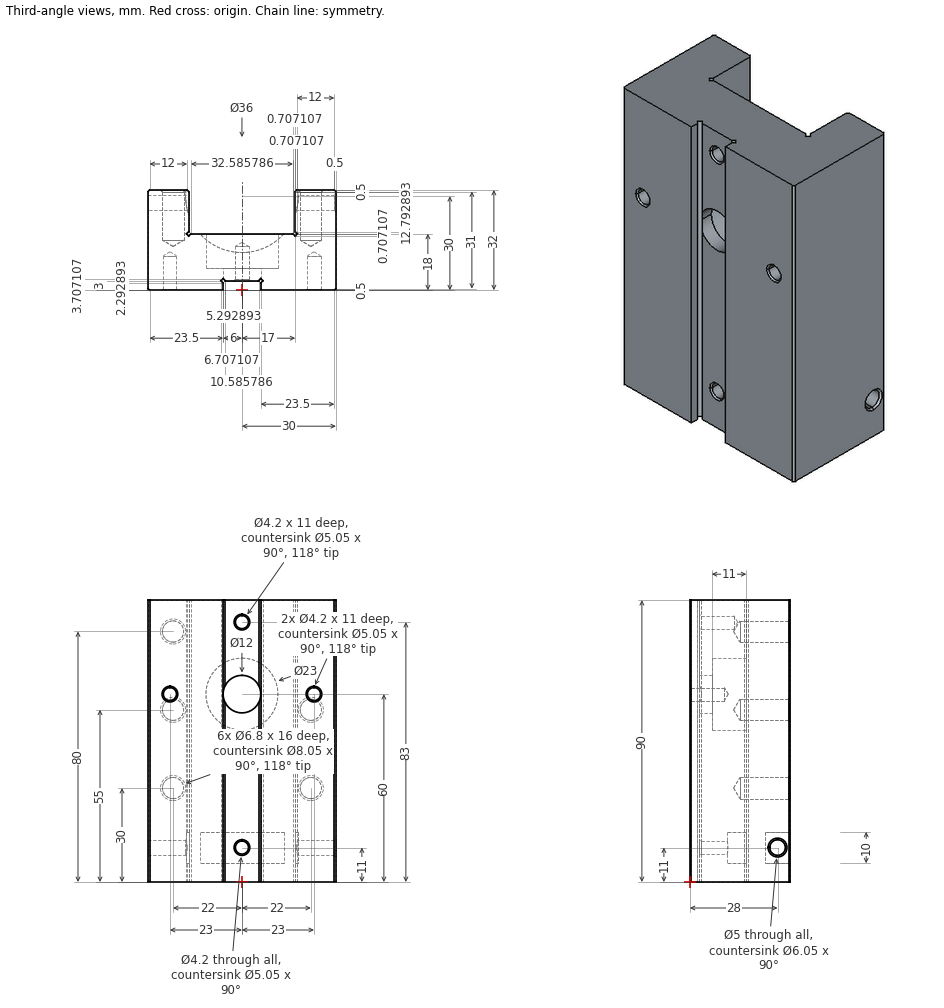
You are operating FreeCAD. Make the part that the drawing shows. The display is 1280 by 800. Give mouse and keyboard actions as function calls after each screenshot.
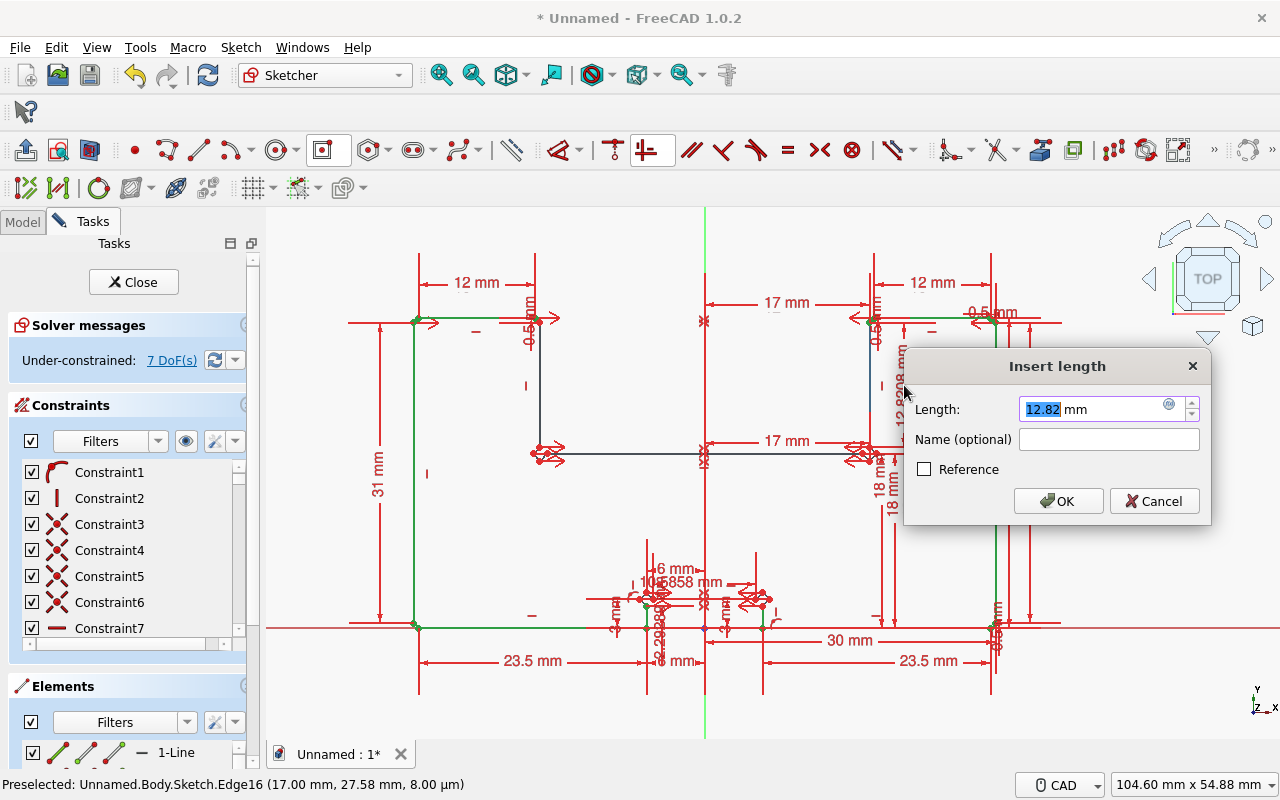
text(12.792893)
key(Return)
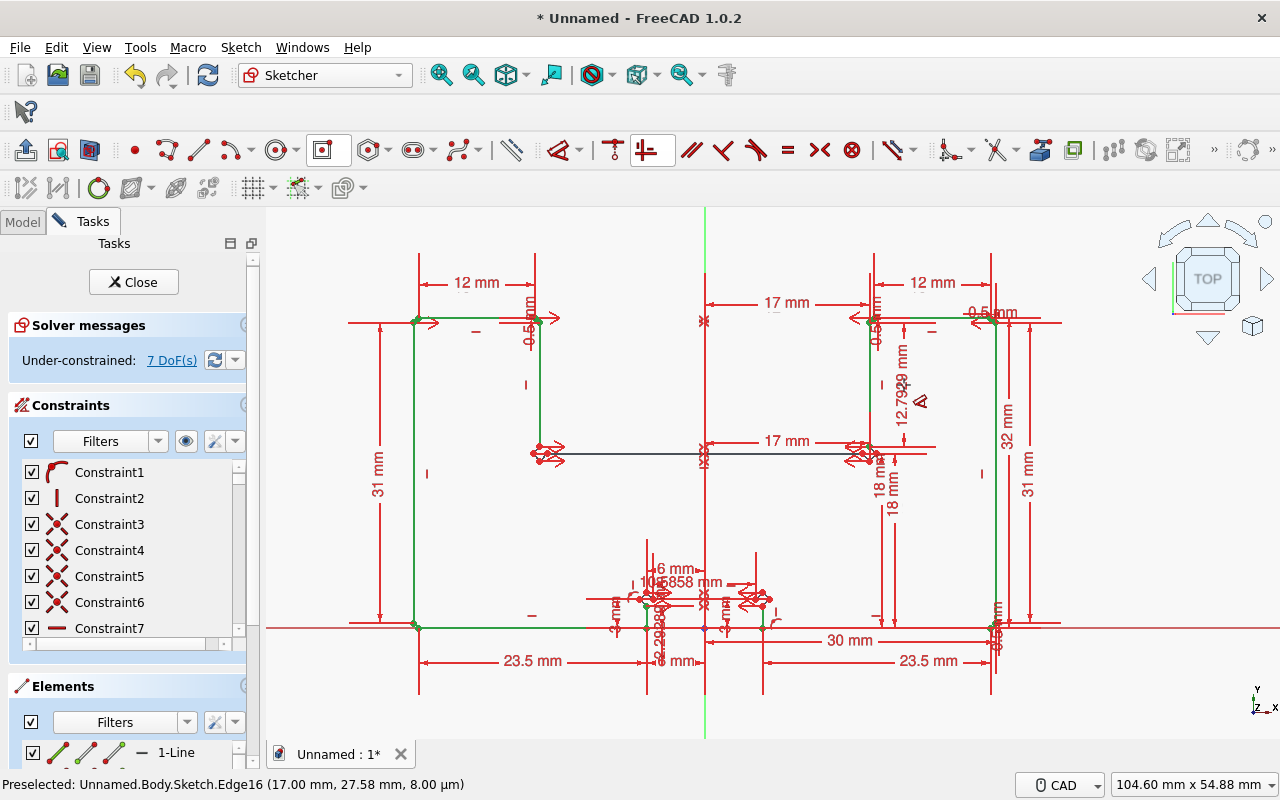
click(768, 454)
click(632, 420)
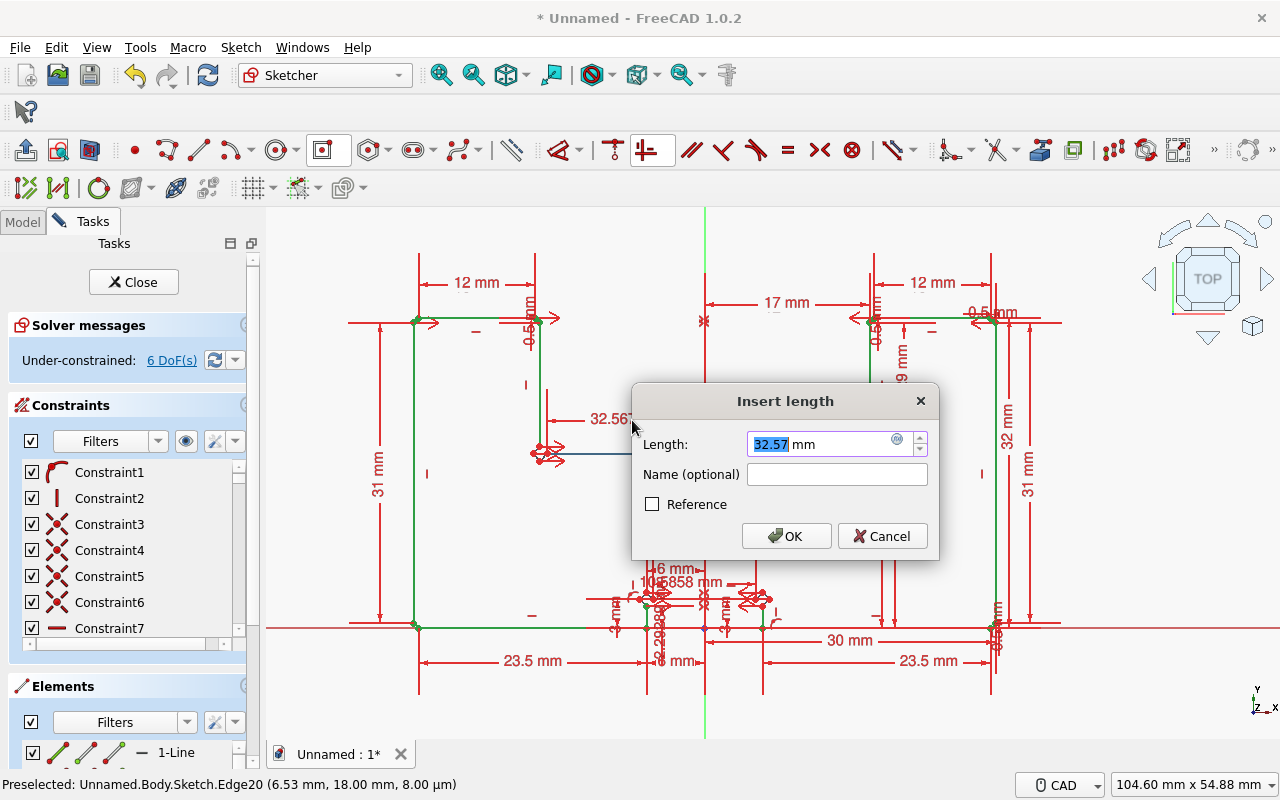
text(32.585786)
key(Return)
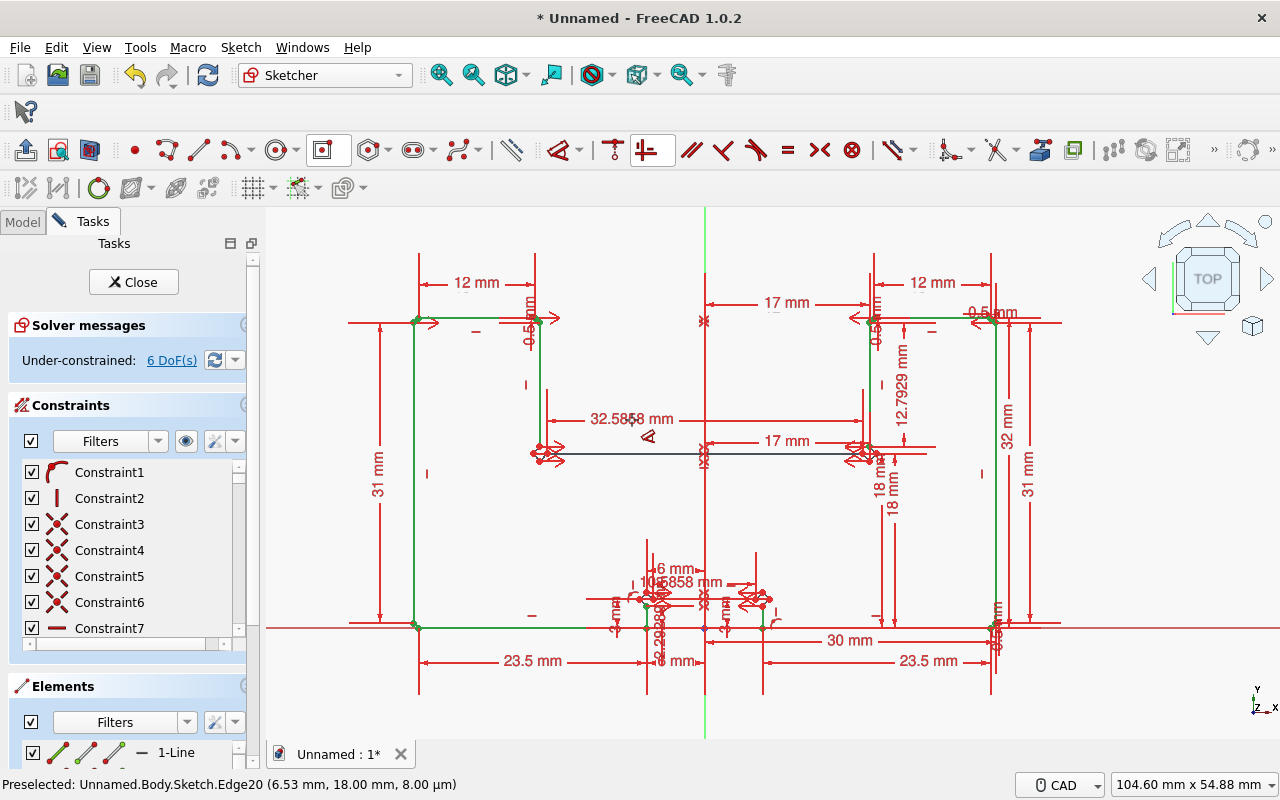
scroll(640, 599, up, 2)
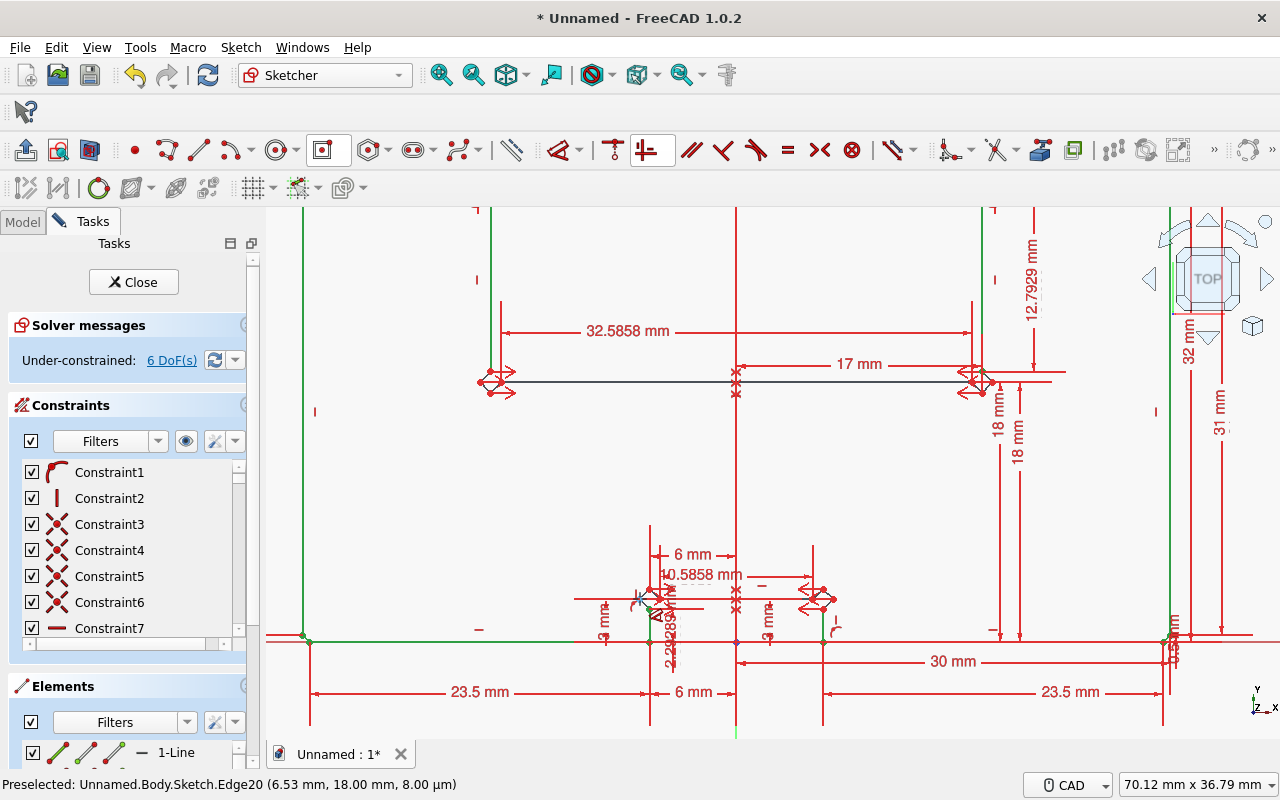
click(640, 599)
click(688, 517)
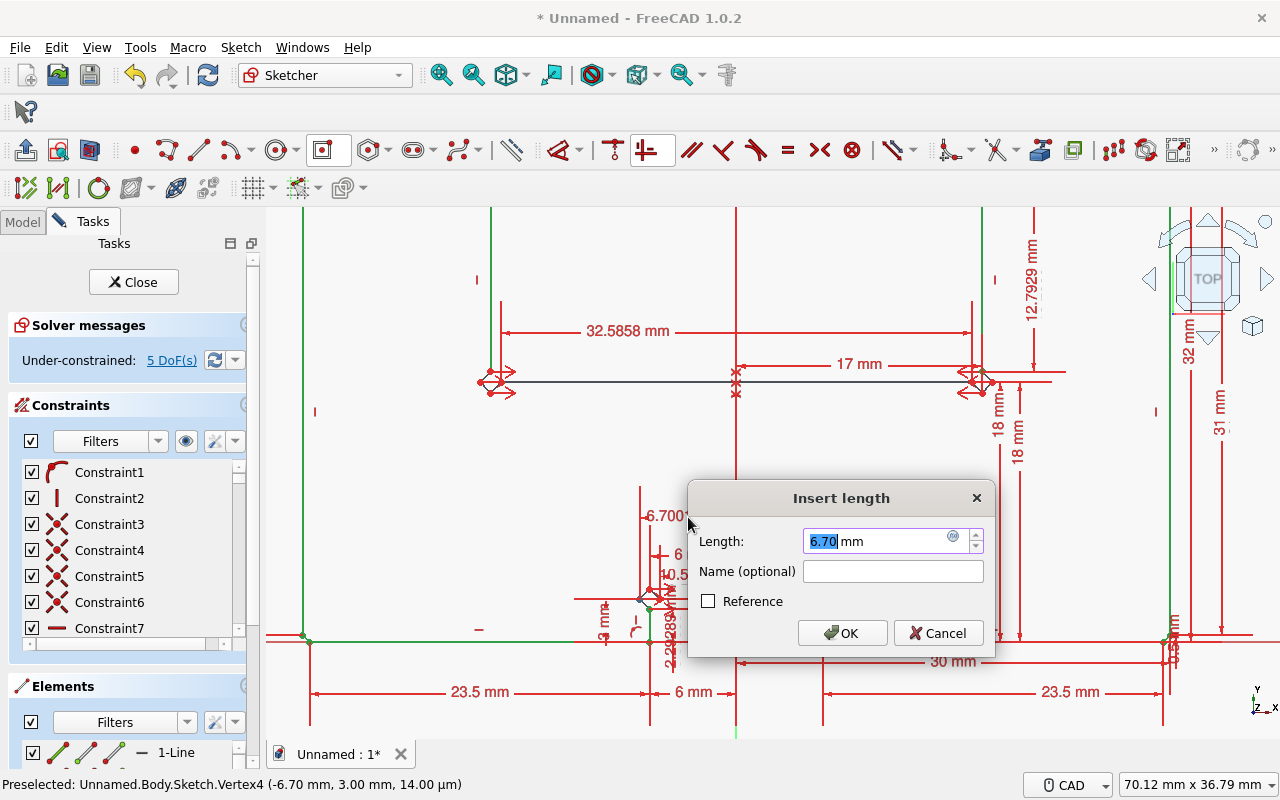
text(6.707107)
key(Return)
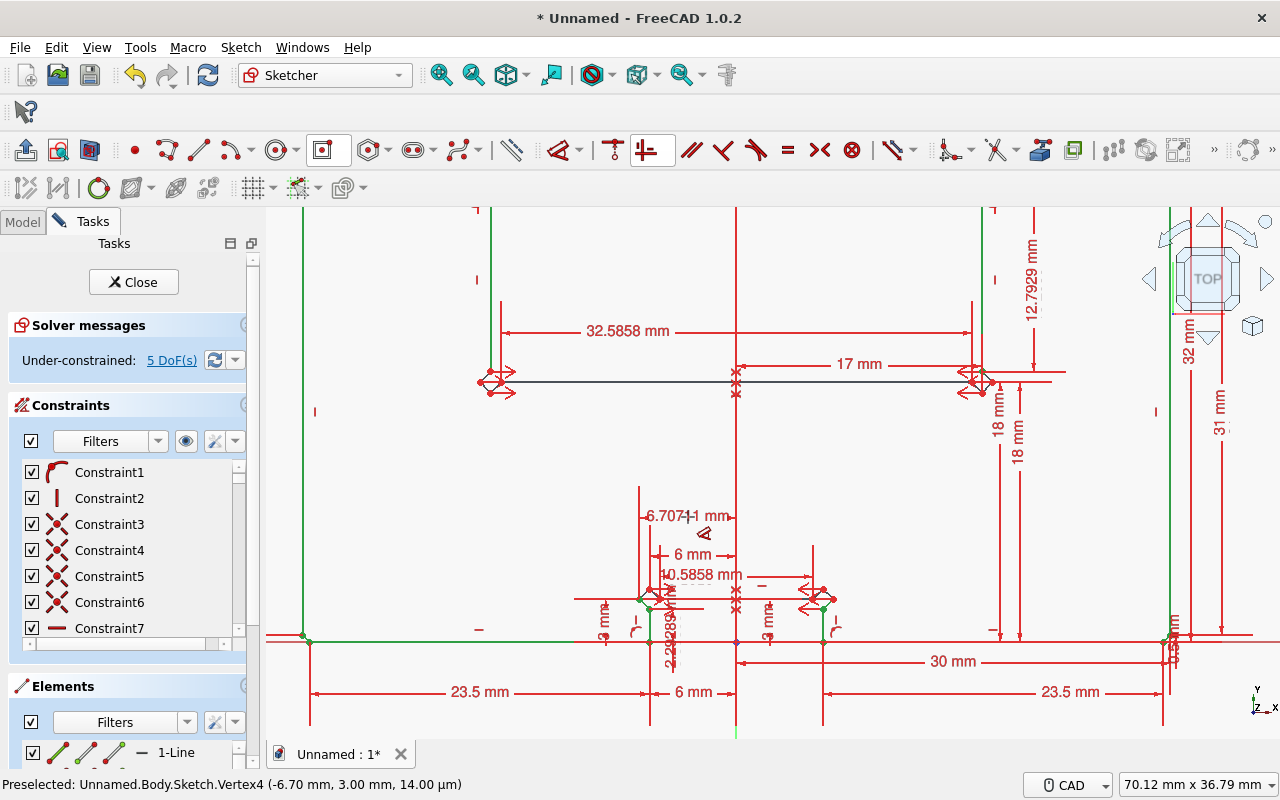
click(650, 589)
click(616, 597)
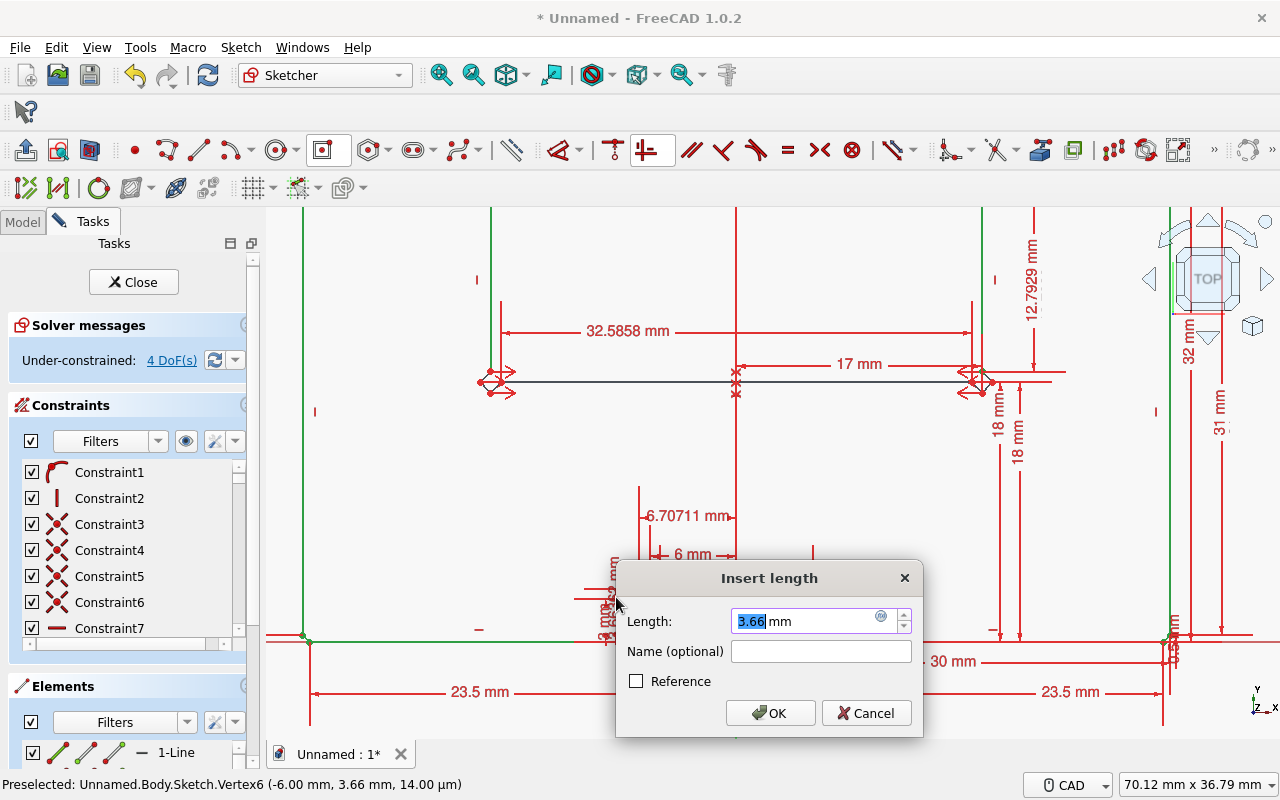
text(3.707107)
key(Return)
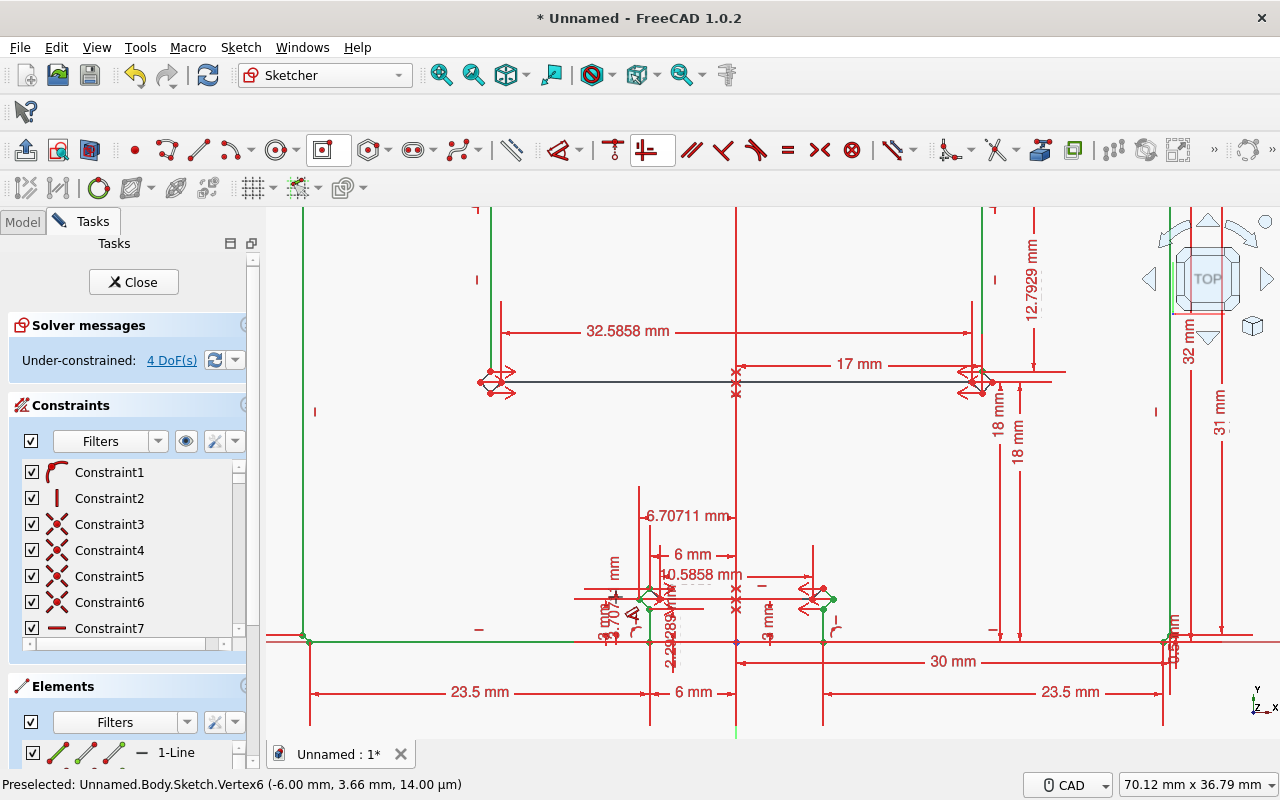
click(660, 599)
click(698, 493)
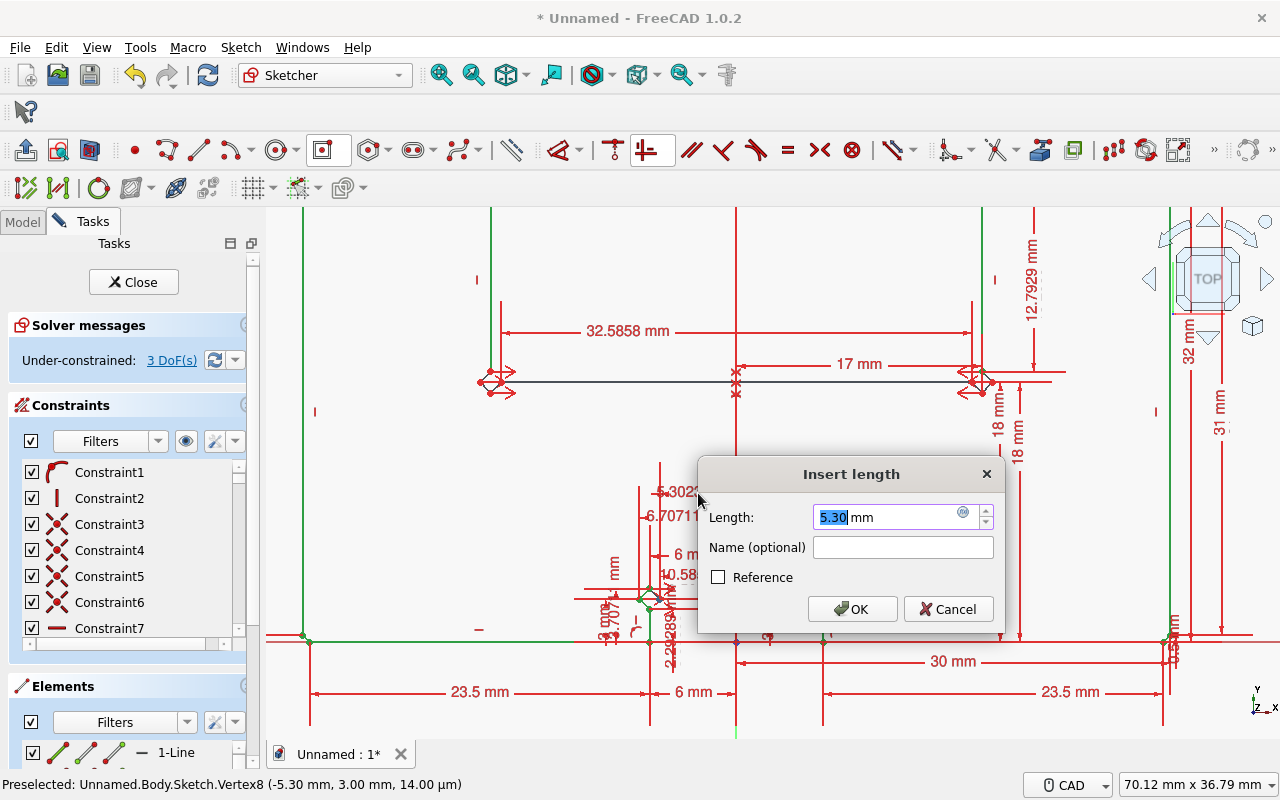
text(5.292893)
key(Return)